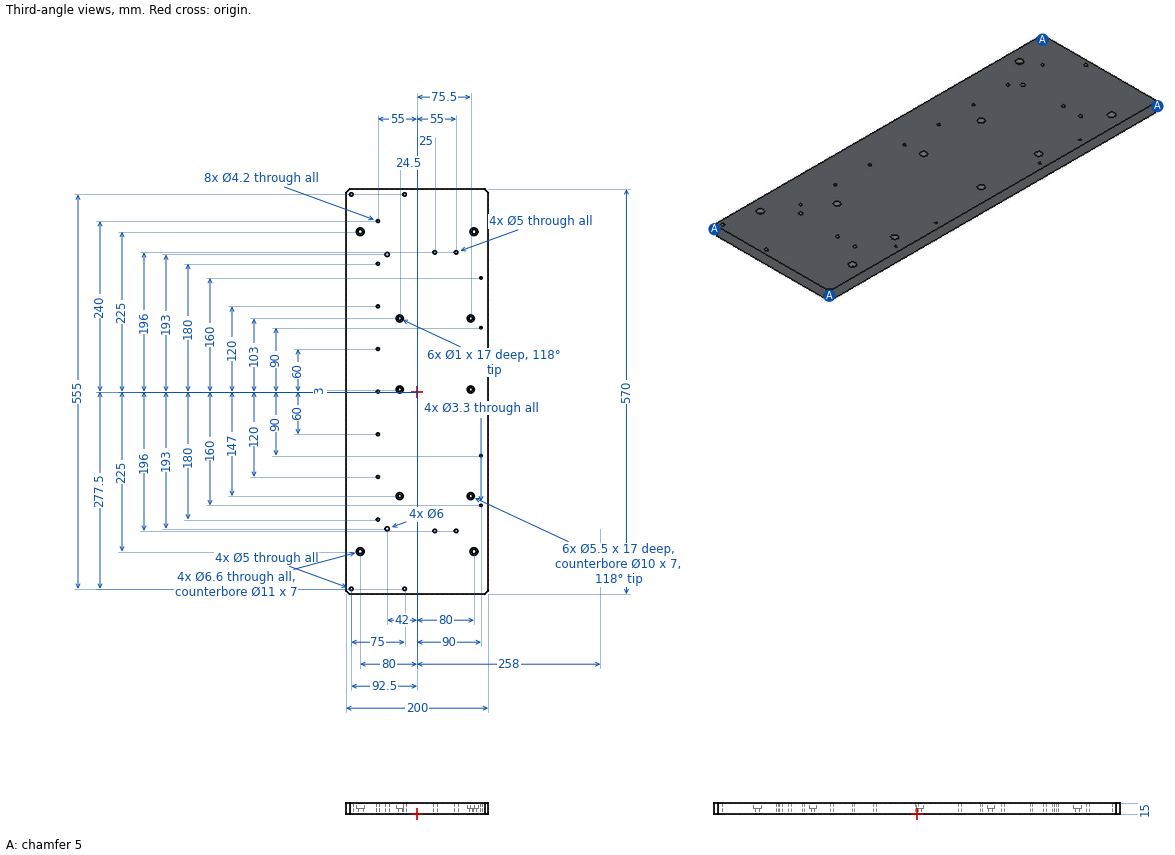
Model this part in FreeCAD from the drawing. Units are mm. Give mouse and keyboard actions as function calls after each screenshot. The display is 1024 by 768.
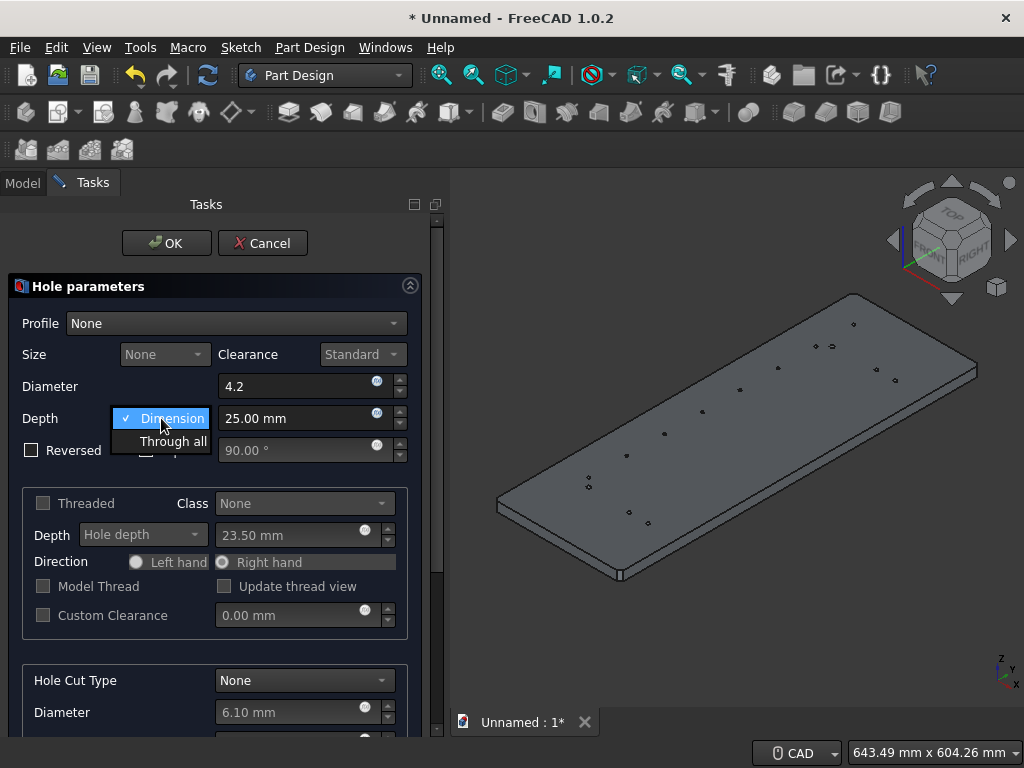
click(160, 442)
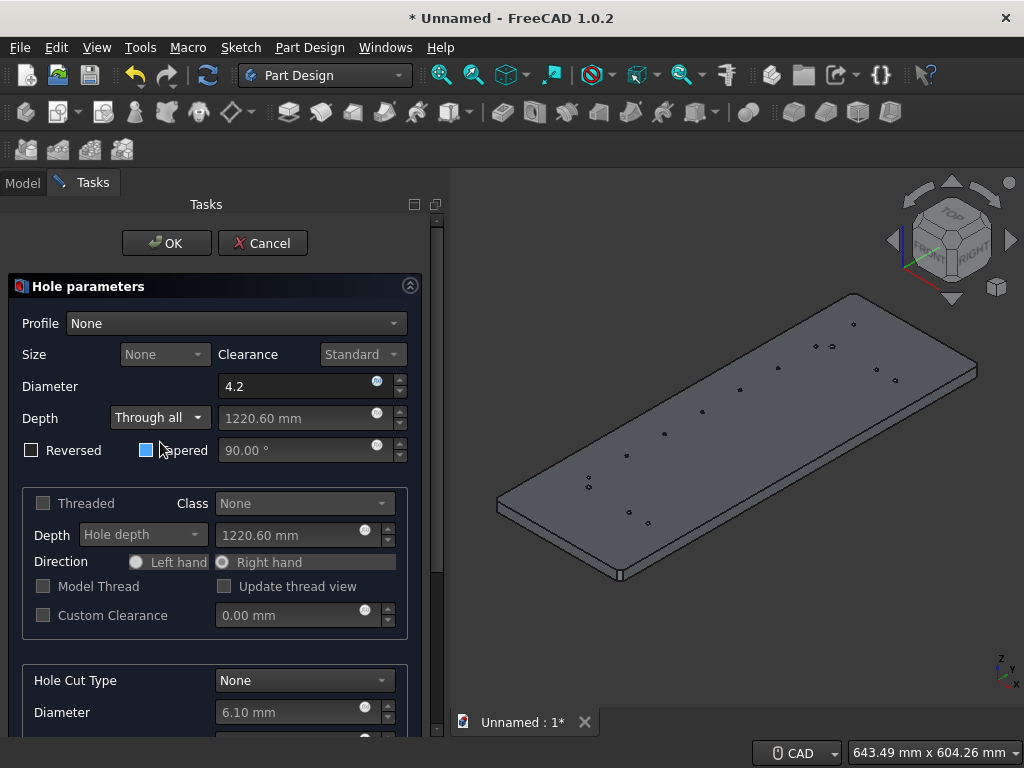
click(167, 243)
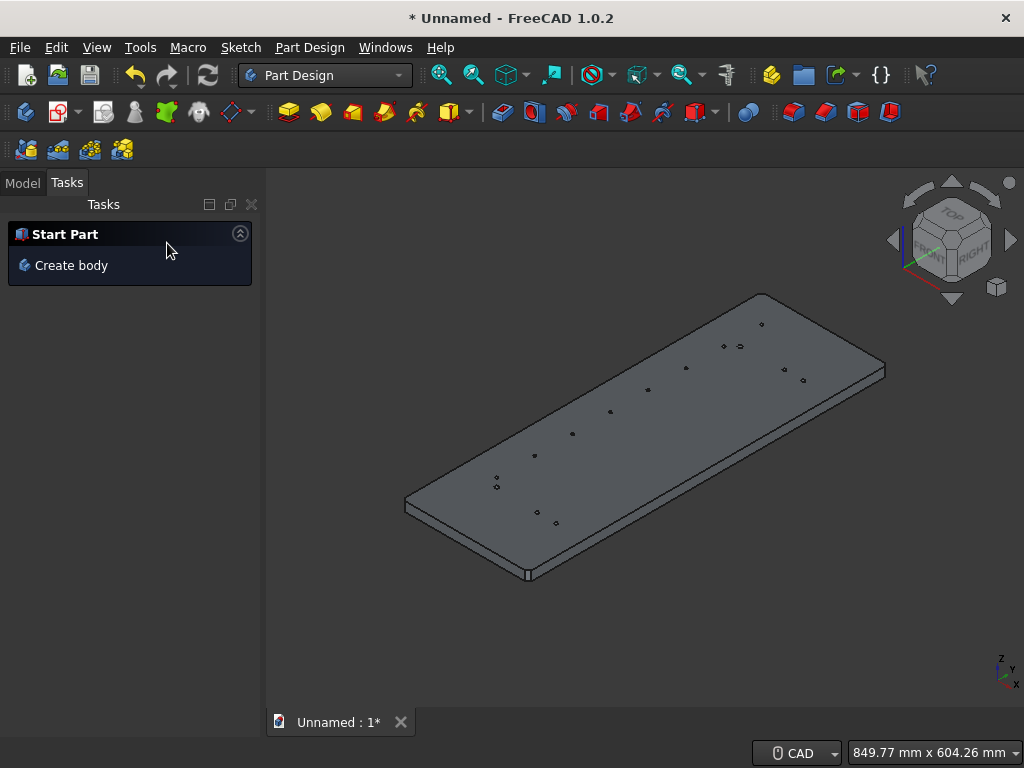
click(714, 412)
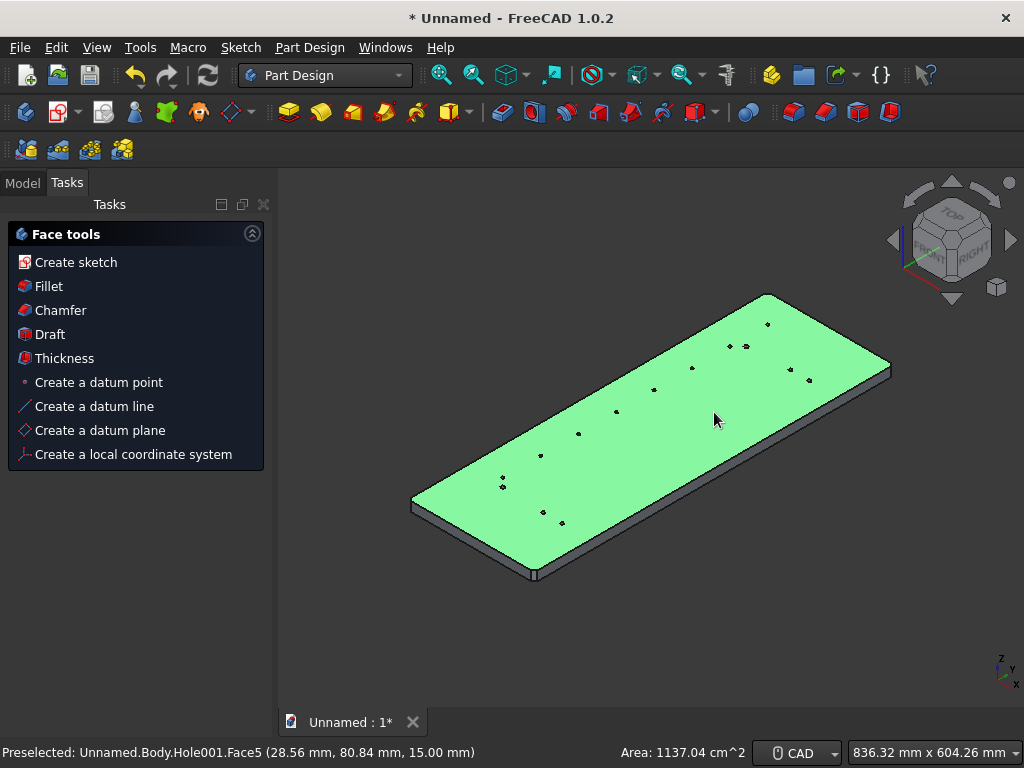
click(58, 112)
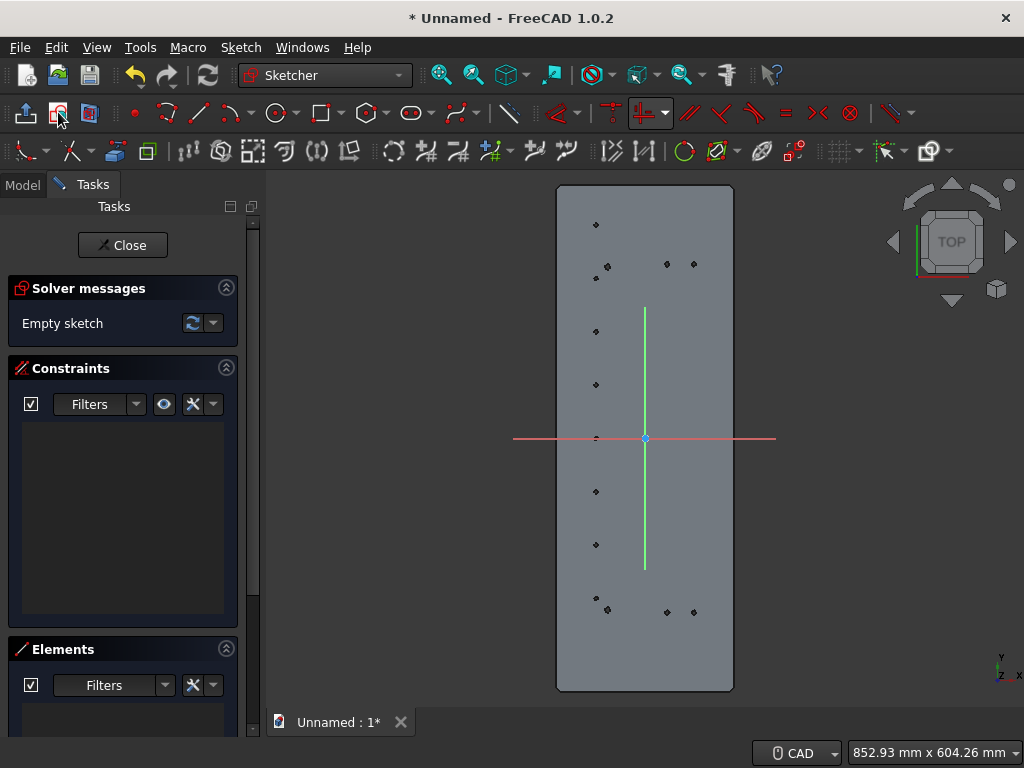
scroll(523, 439, down, 2)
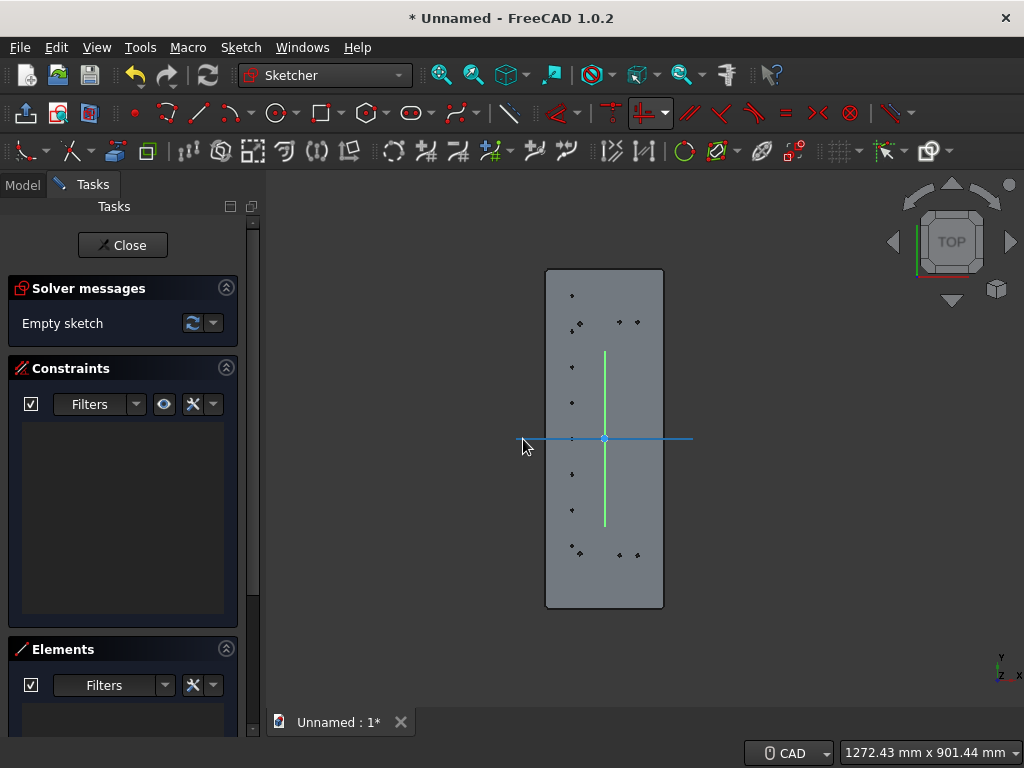
click(276, 114)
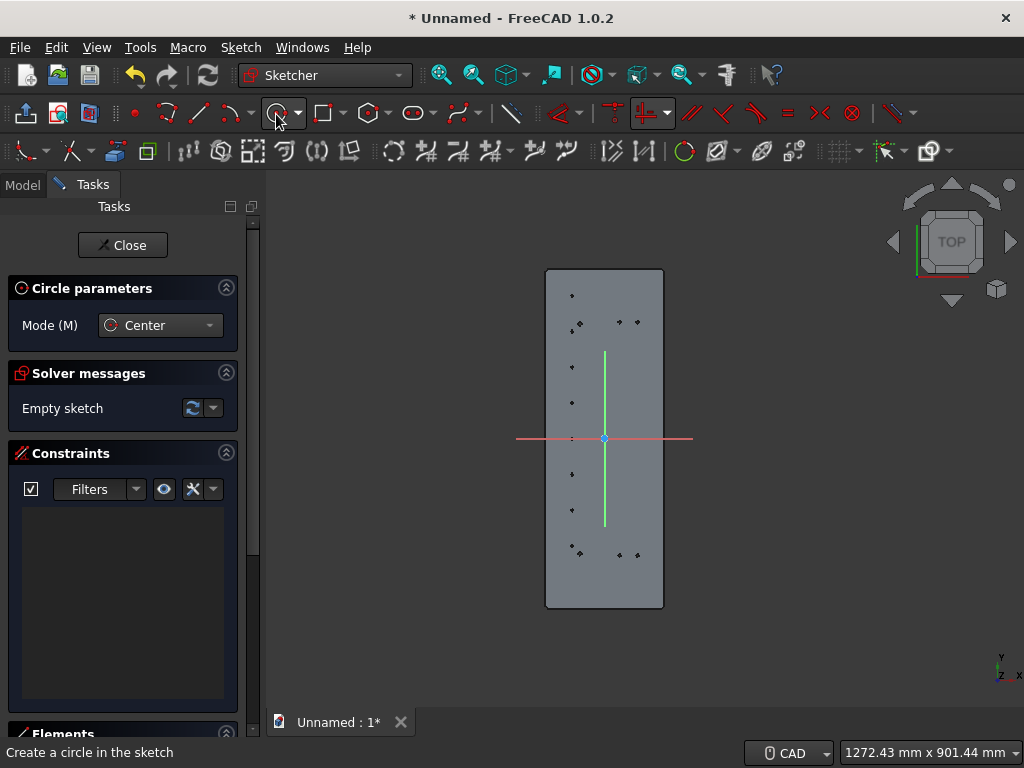
scroll(550, 604, up, 14)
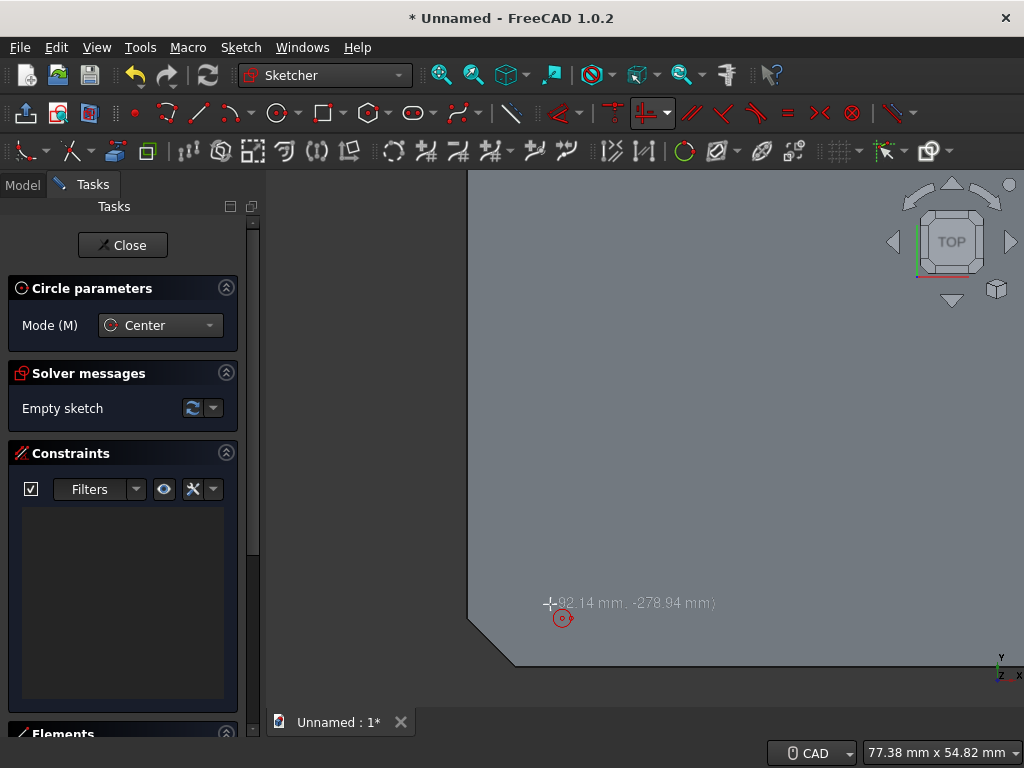
scroll(550, 604, down, 14)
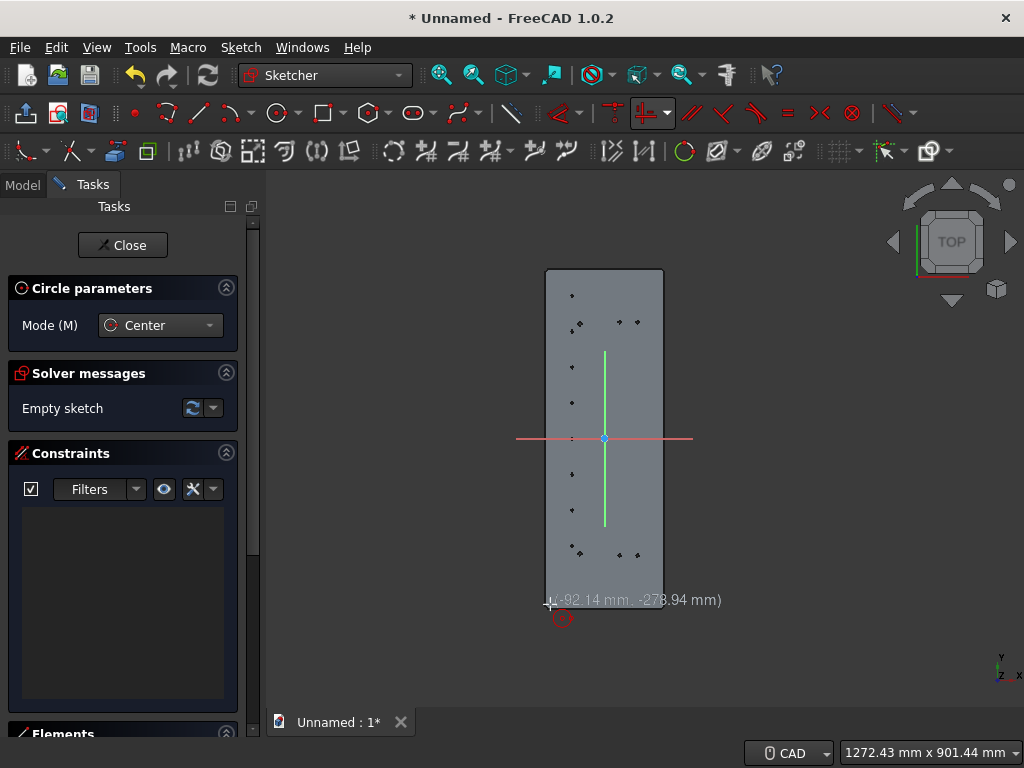
click(550, 604)
move(551, 603)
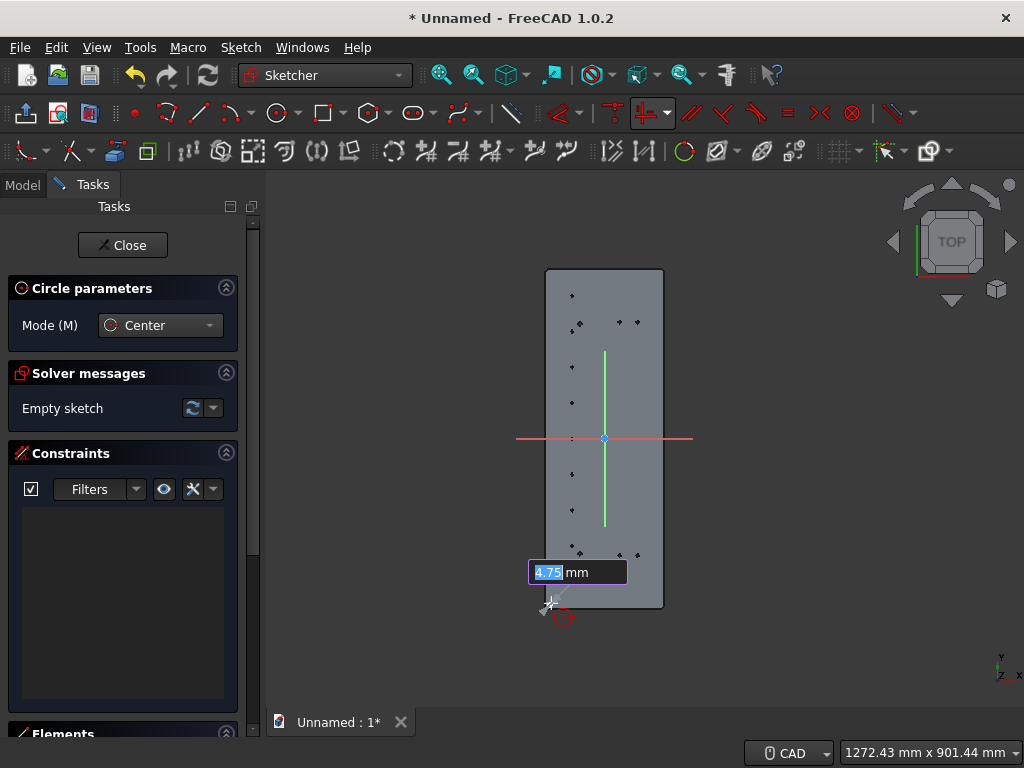
text(5)
key(Return)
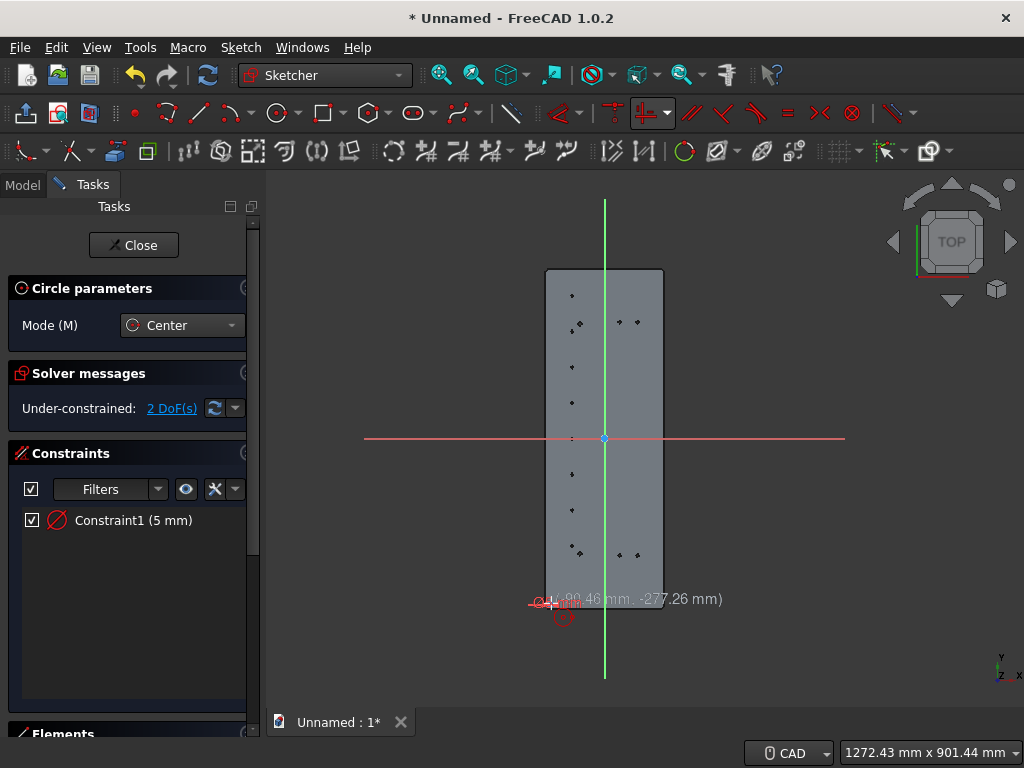
scroll(594, 604, up, 14)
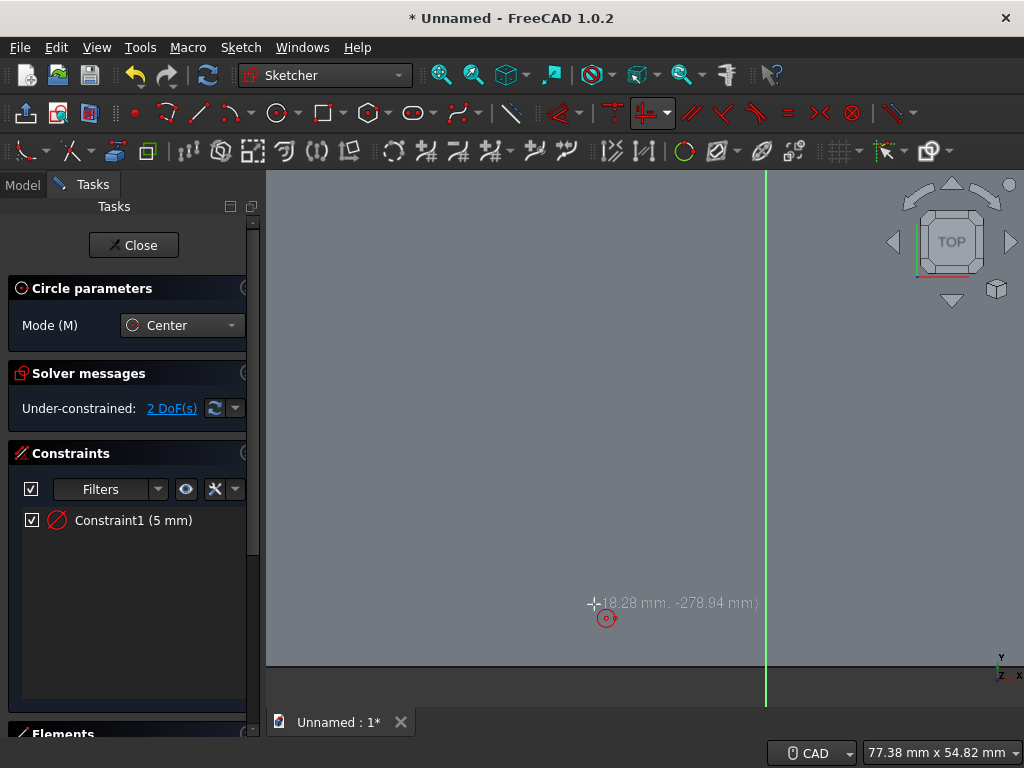
scroll(594, 604, down, 14)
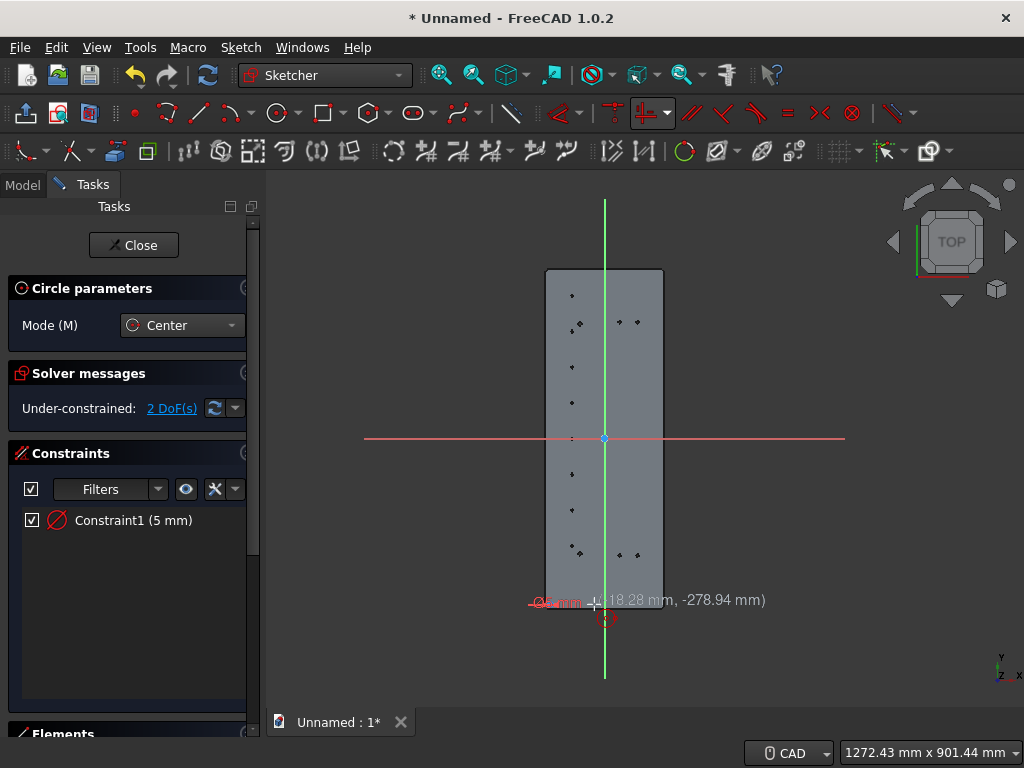
scroll(594, 604, up, 3)